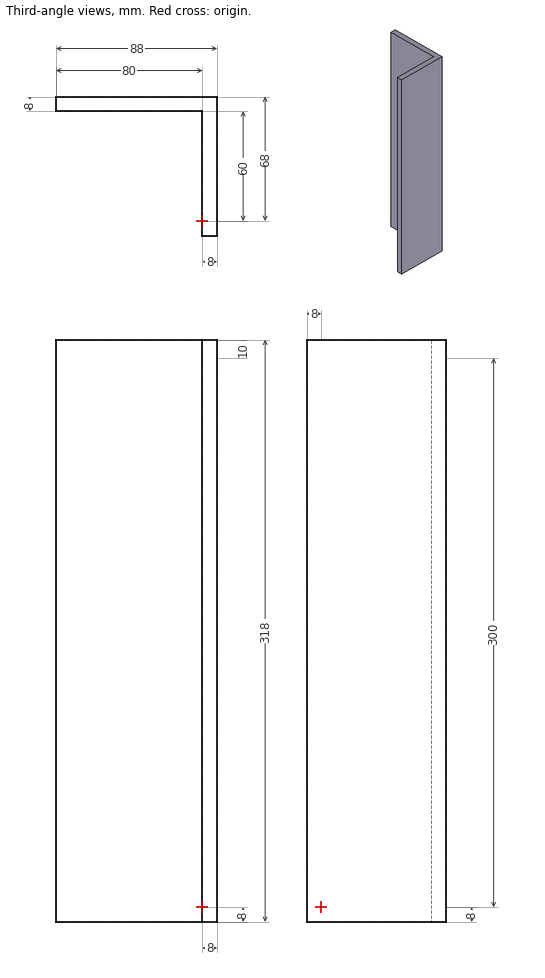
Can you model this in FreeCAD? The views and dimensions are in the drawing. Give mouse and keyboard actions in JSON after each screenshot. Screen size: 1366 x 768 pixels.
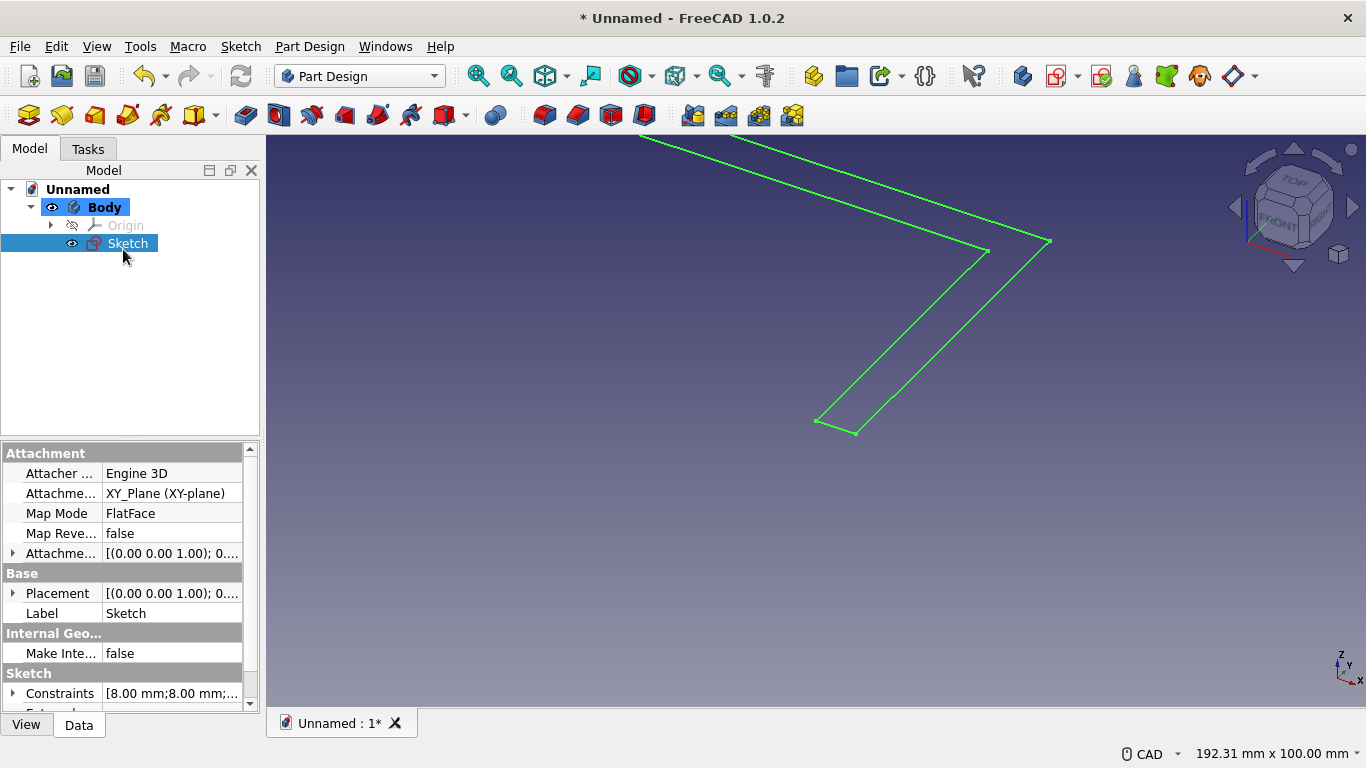
{"action": "left_click", "coordinate": [29, 116]}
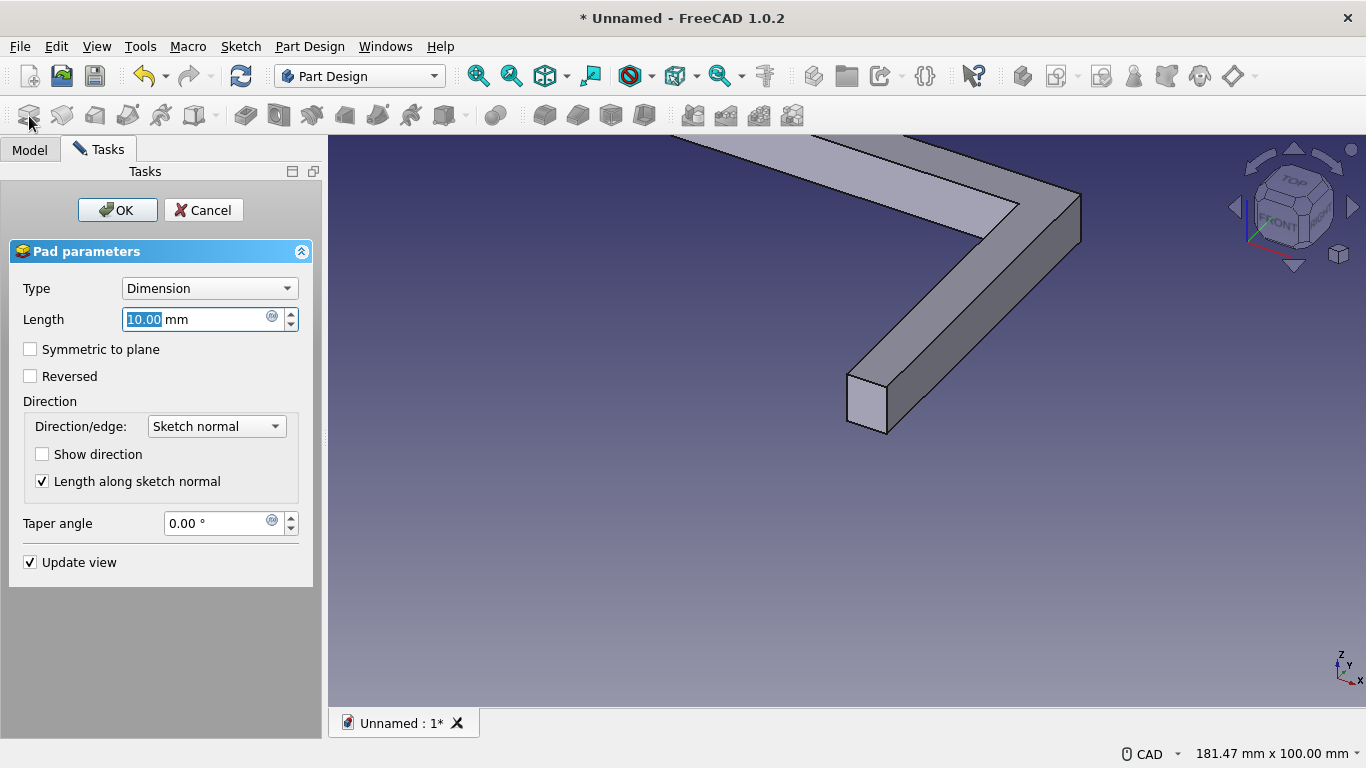
{"action": "type", "text": "300"}
{"action": "key", "text": "Tab"}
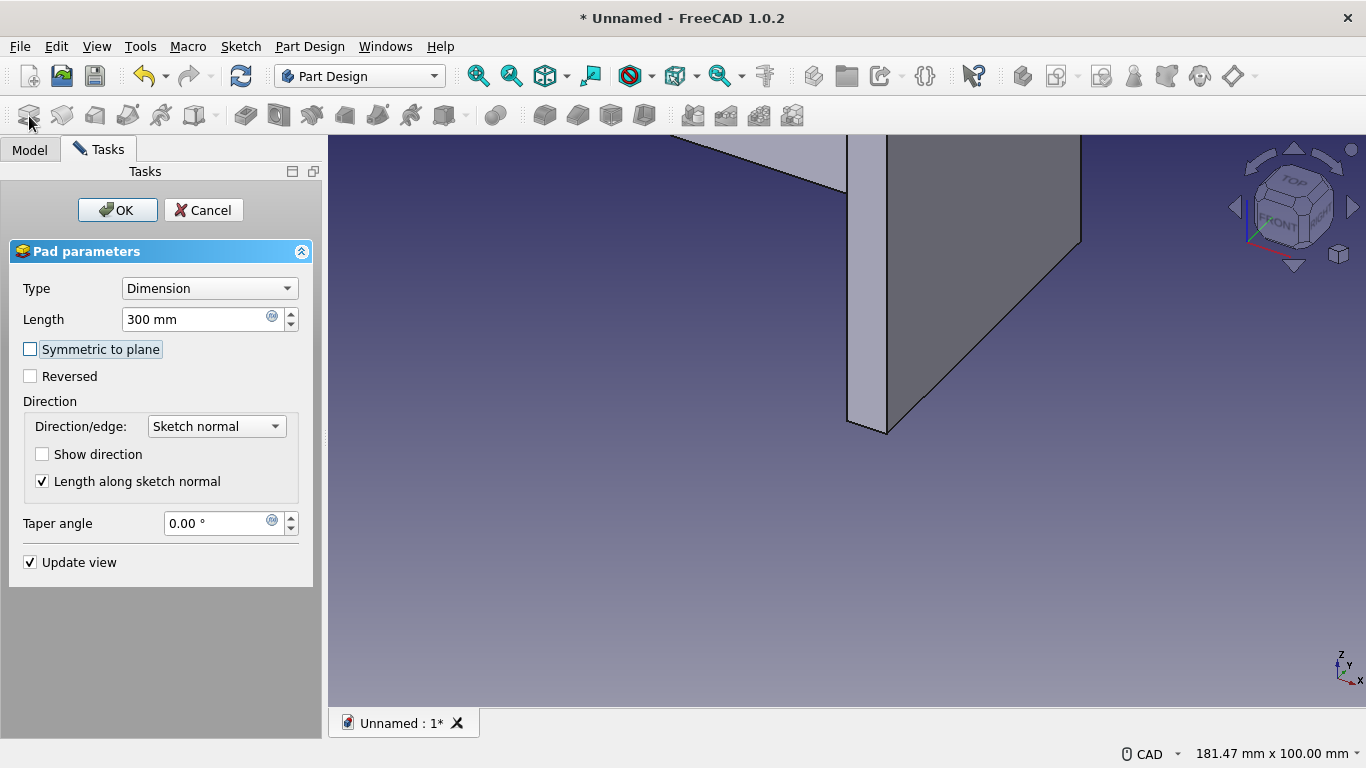
{"action": "left_click", "coordinate": [118, 210]}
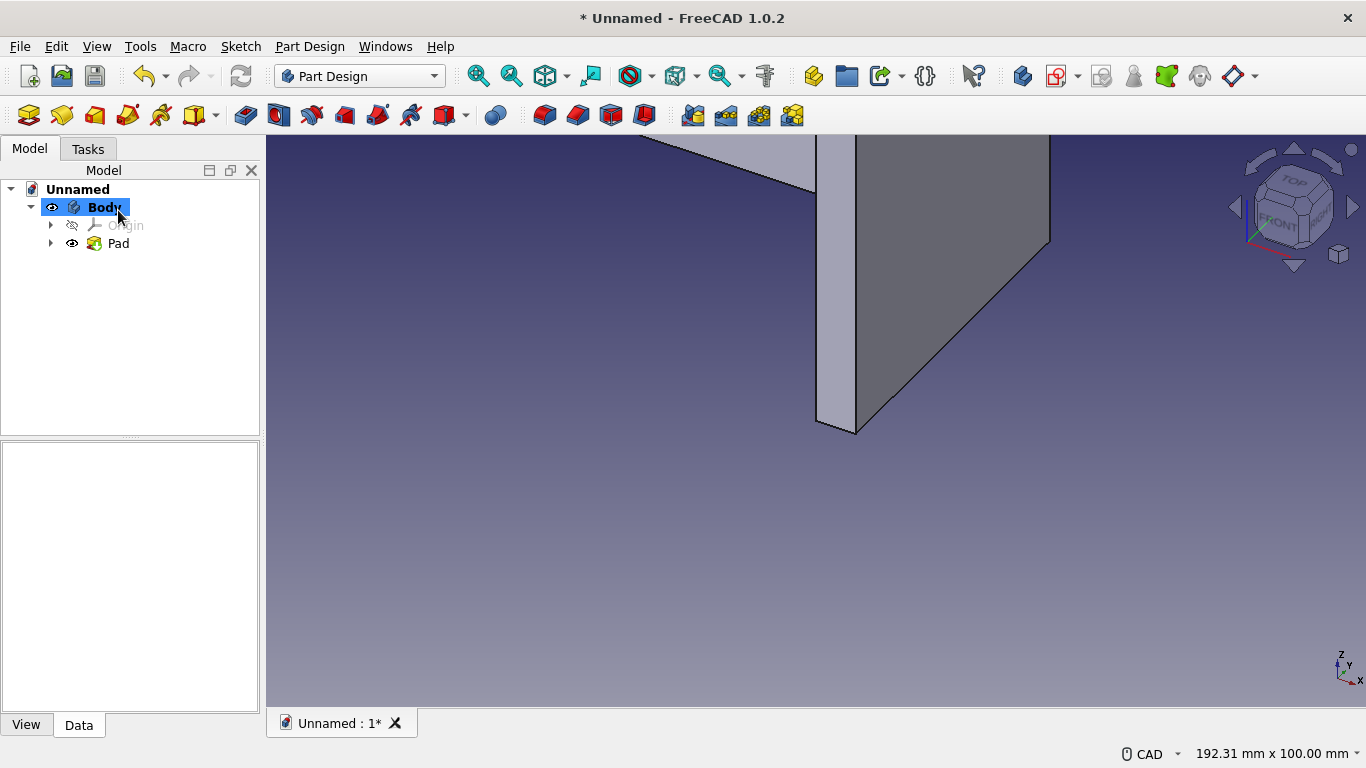
{"action": "left_click", "coordinate": [479, 76]}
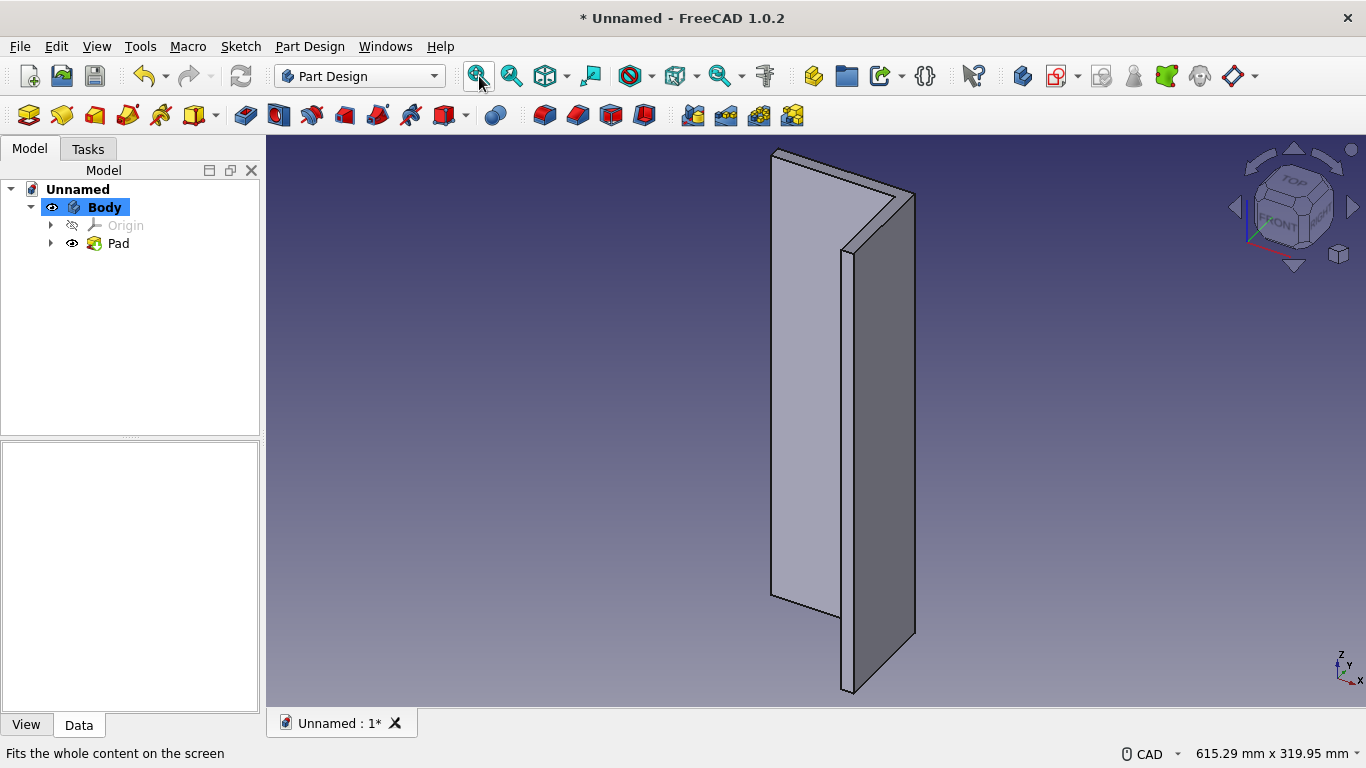
{"action": "left_click", "coordinate": [900, 194]}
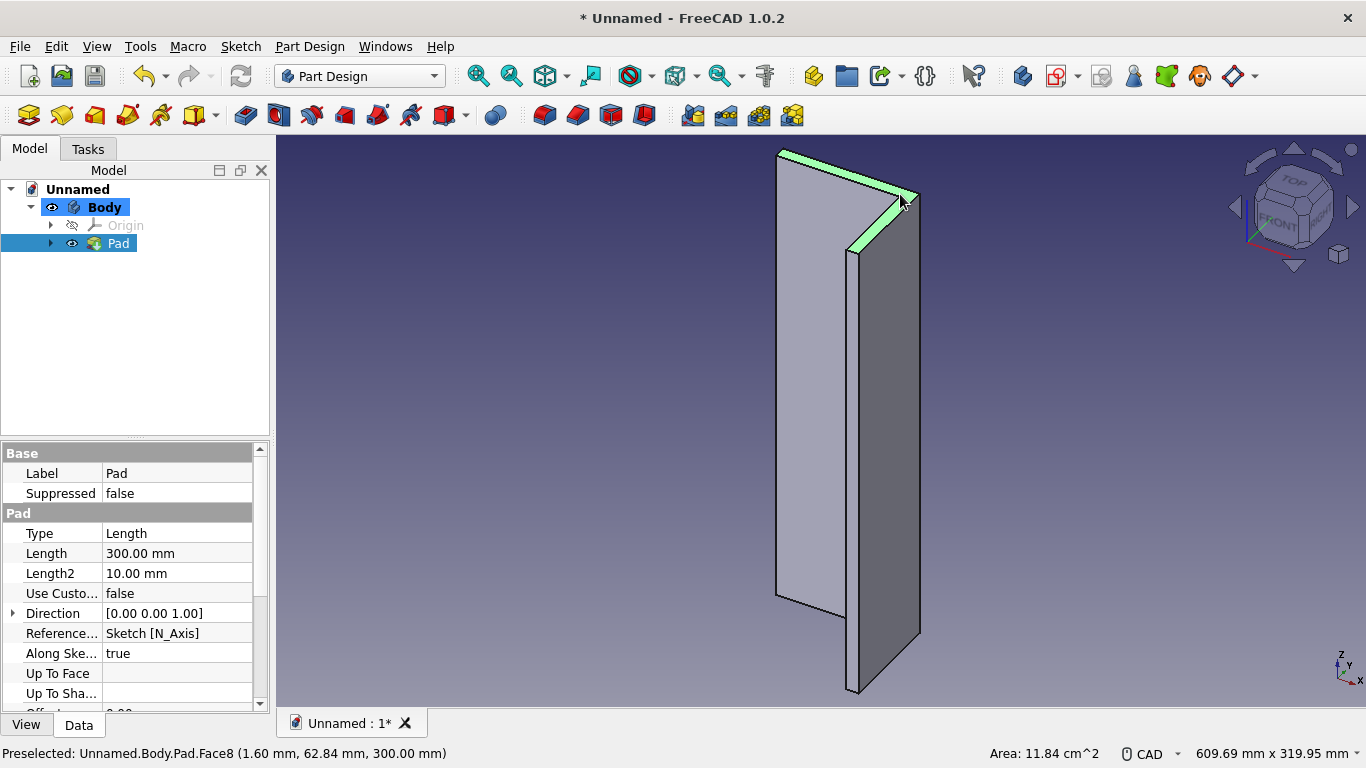
{"action": "left_click", "coordinate": [1056, 76]}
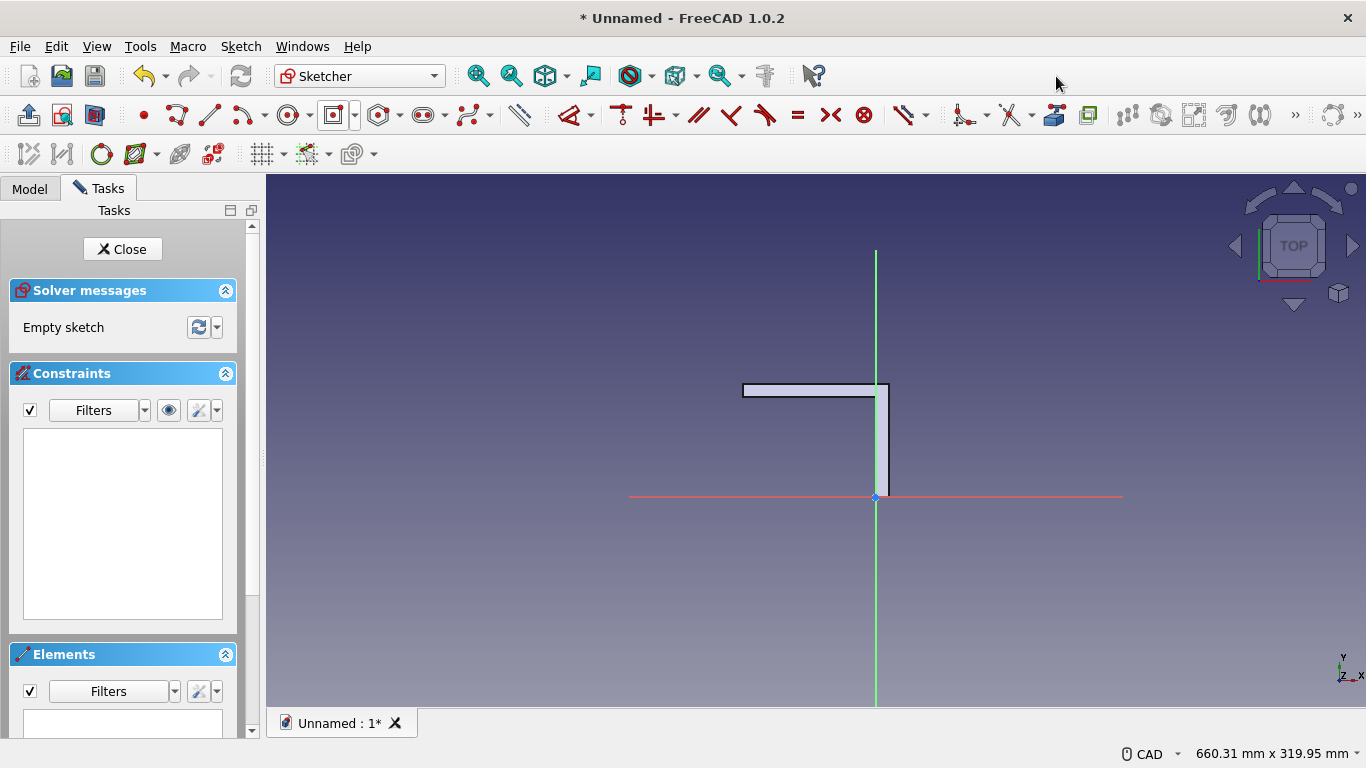
{"action": "scroll", "coordinate": [856, 440], "scroll_direction": "up", "scroll_amount": 5}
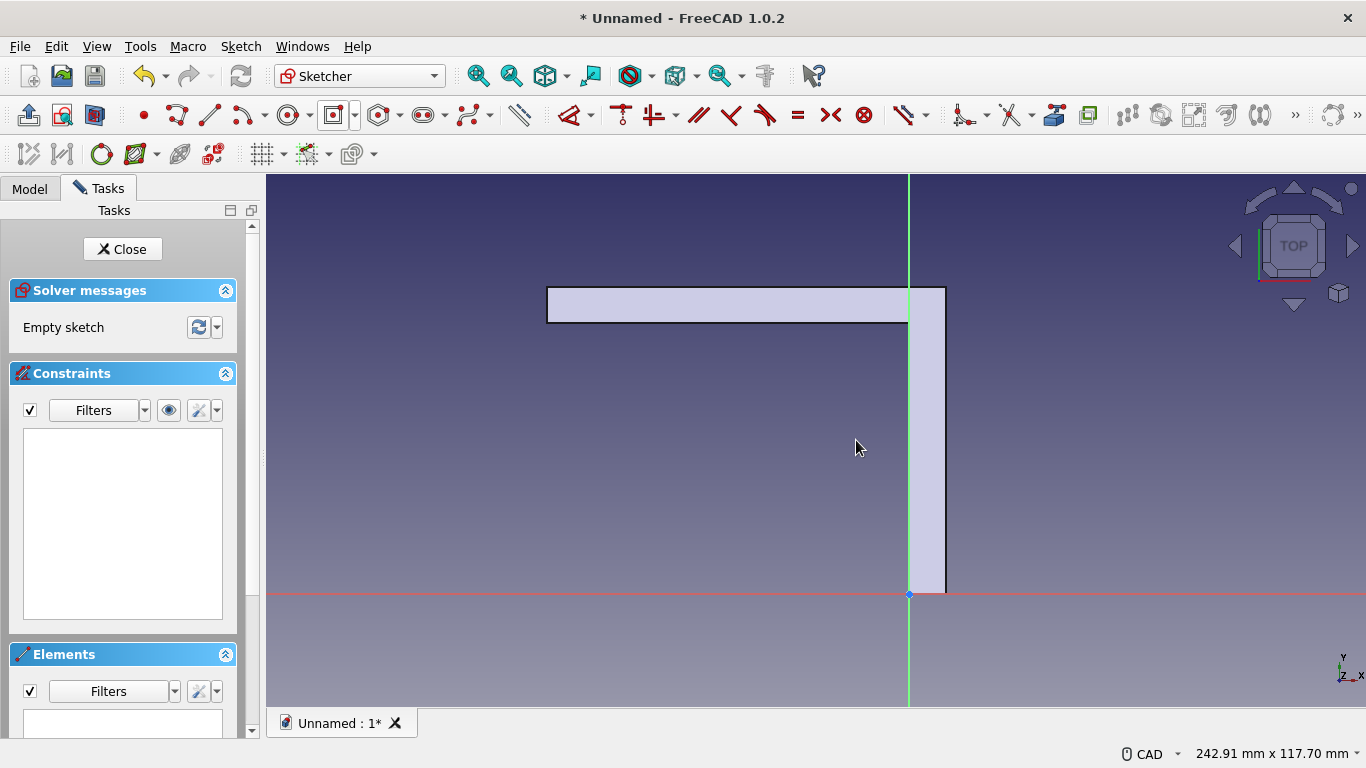
{"action": "left_click", "coordinate": [177, 116]}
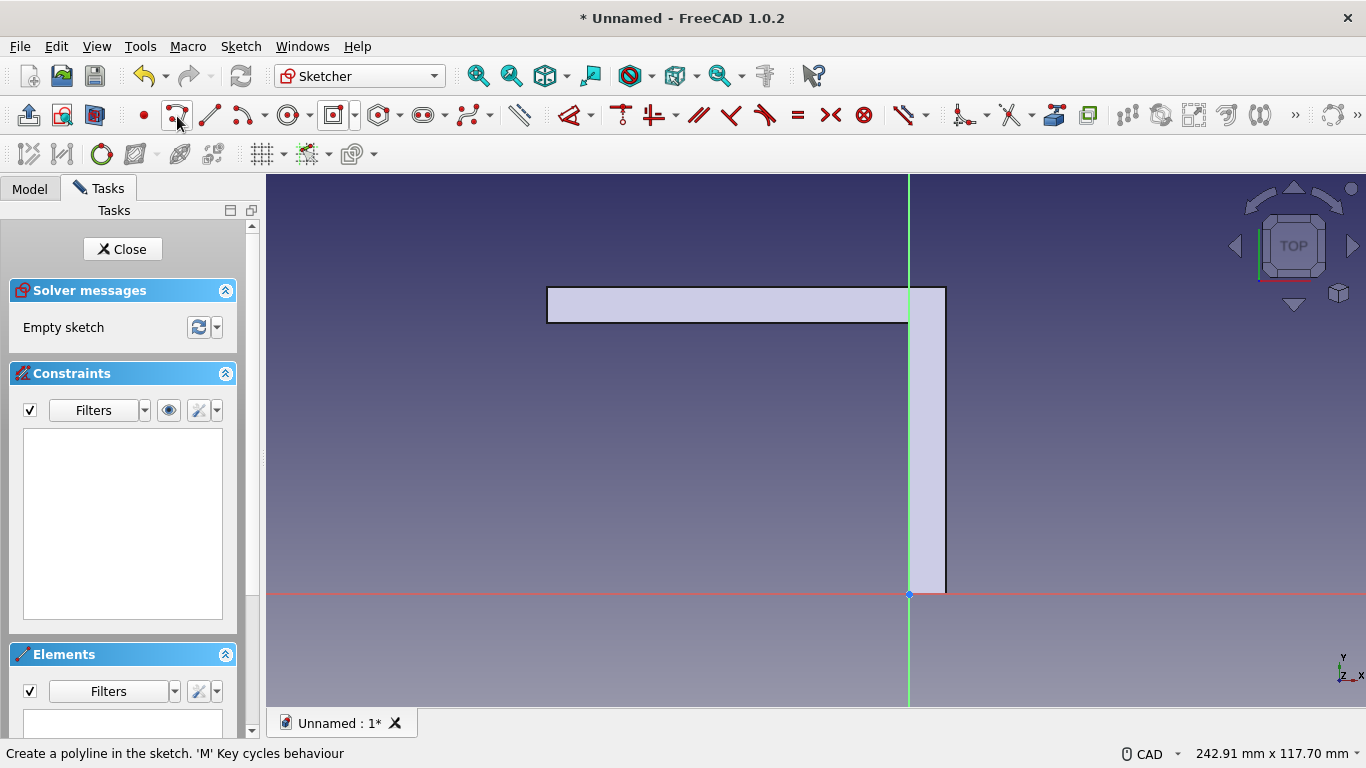
{"action": "left_click", "coordinate": [909, 594]}
{"action": "left_click", "coordinate": [946, 585]}
{"action": "left_click", "coordinate": [946, 287]}
{"action": "left_click", "coordinate": [547, 287]}
{"action": "left_click", "coordinate": [547, 323]}
{"action": "left_click", "coordinate": [900, 323]}
{"action": "left_click", "coordinate": [909, 594]}
{"action": "key", "text": "Escape"}
{"action": "key", "text": "Escape"}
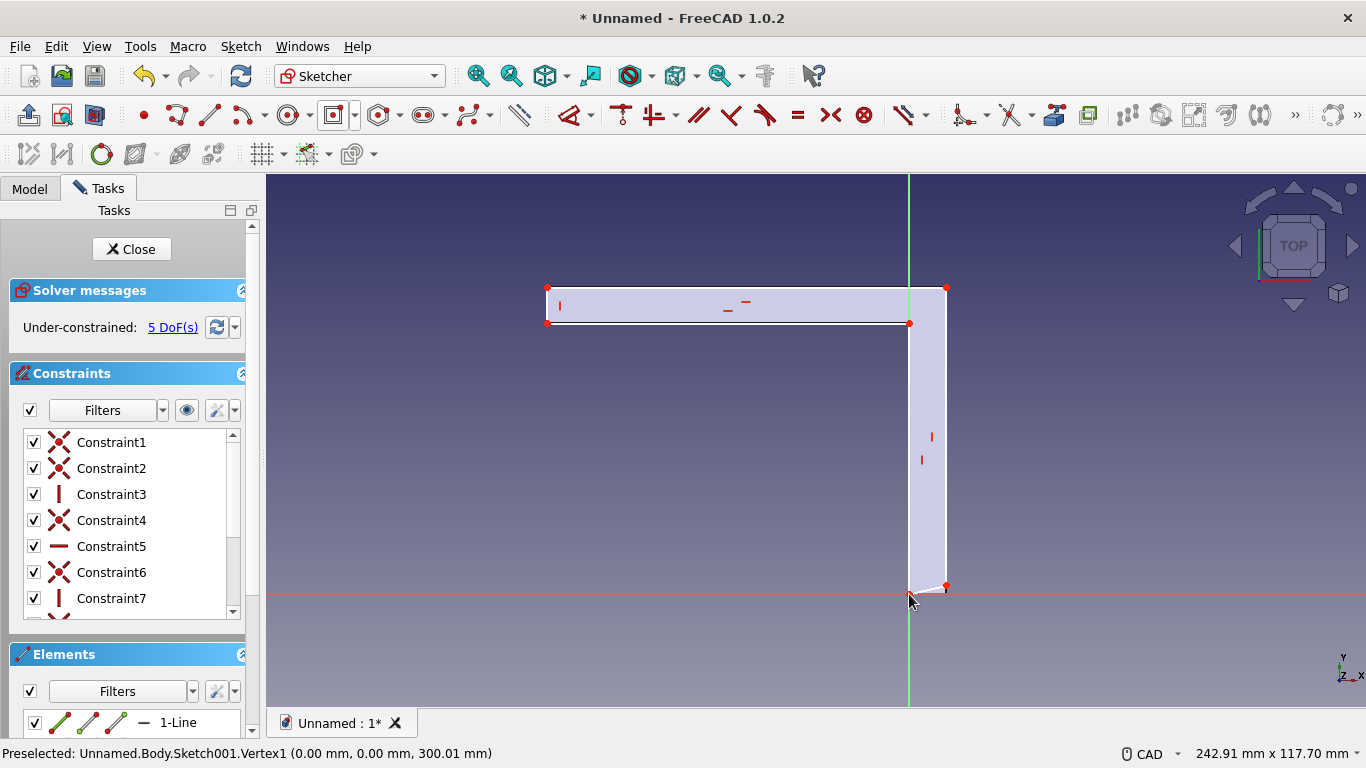
{"action": "scroll", "coordinate": [920, 592], "scroll_direction": "up", "scroll_amount": 2}